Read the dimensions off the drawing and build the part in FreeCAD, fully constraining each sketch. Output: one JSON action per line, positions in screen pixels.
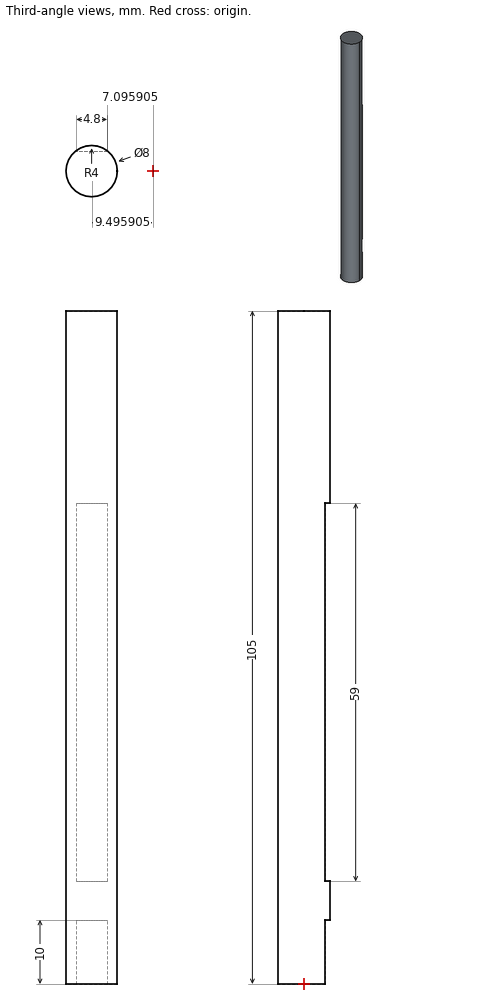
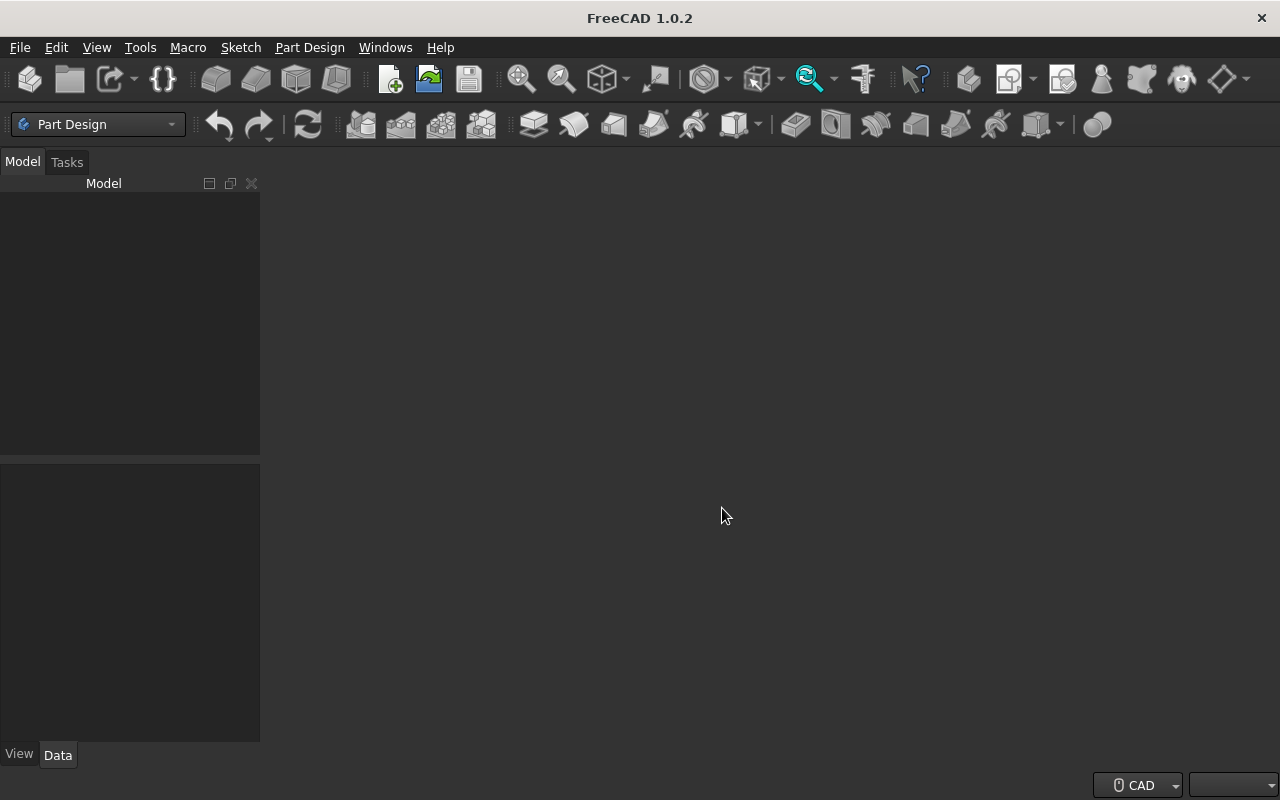
{"action": "left_click", "coordinate": [390, 80]}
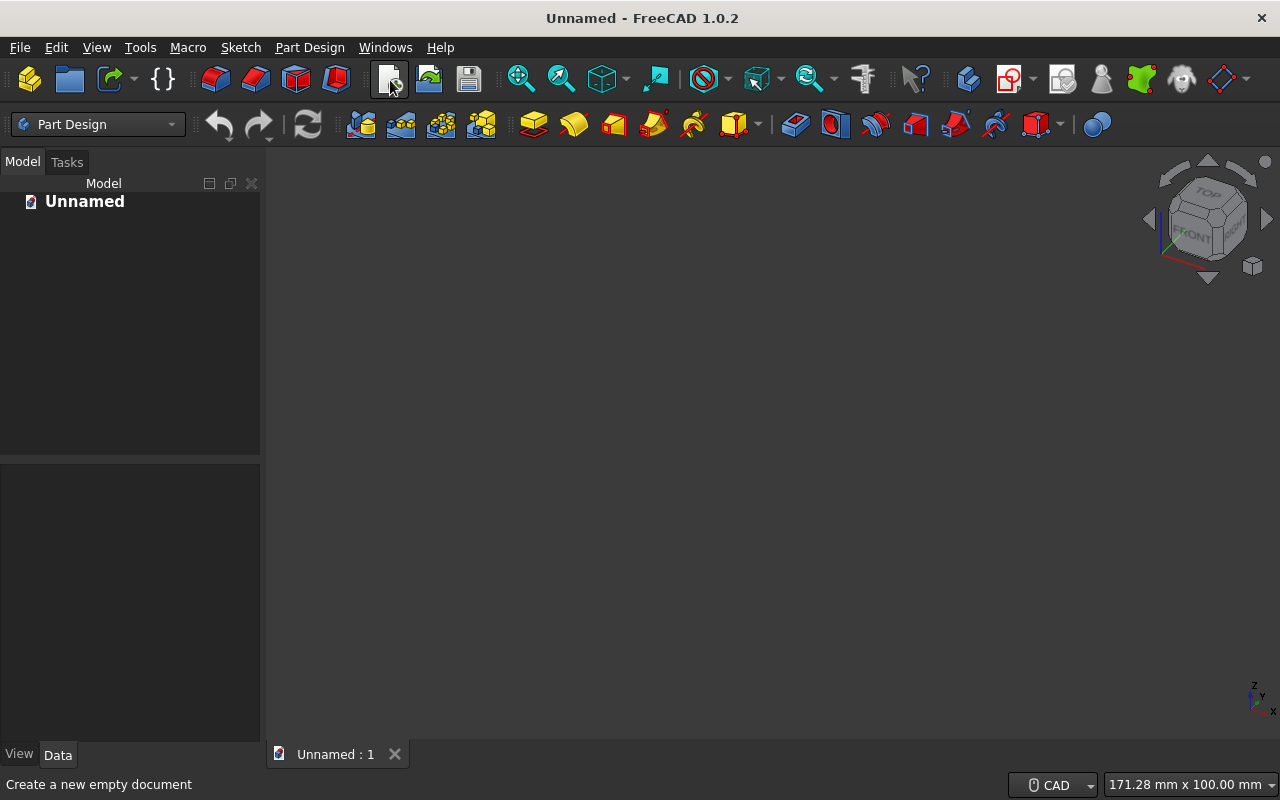
{"action": "left_click", "coordinate": [1010, 80]}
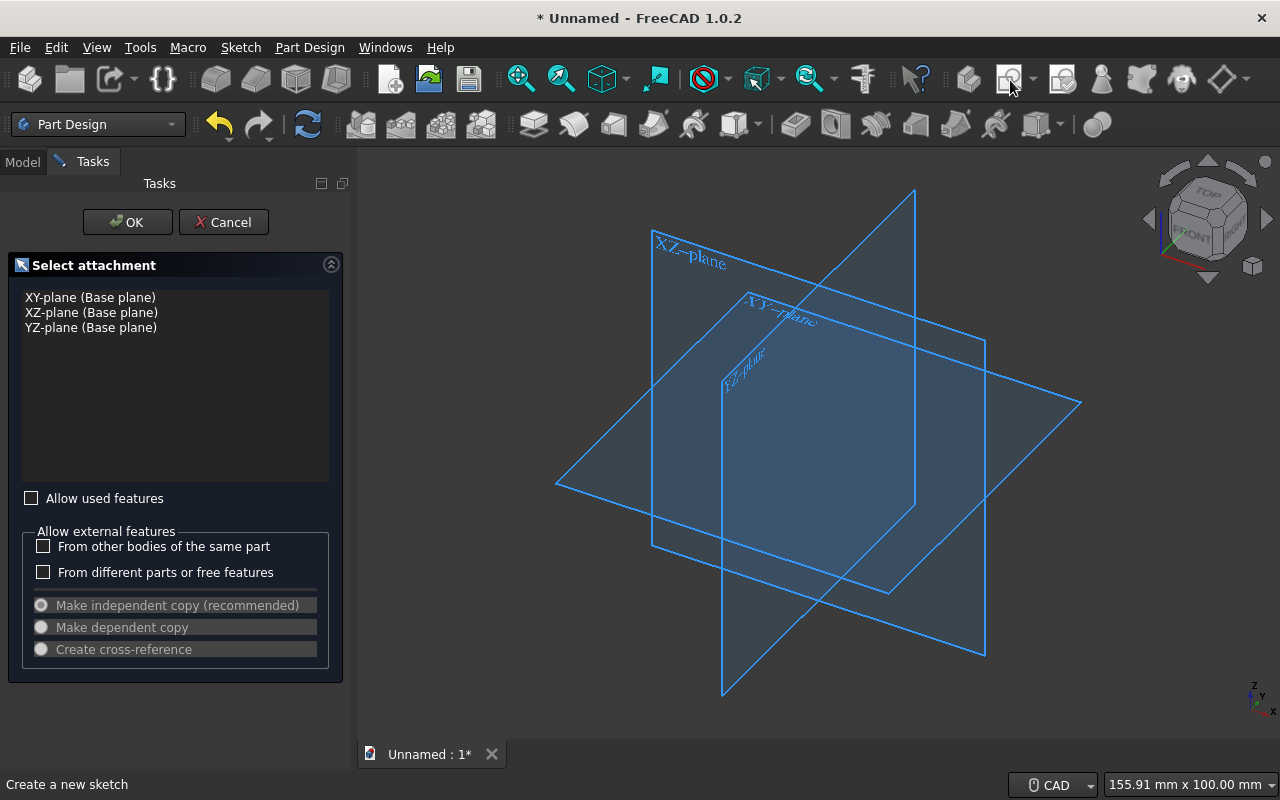
{"action": "left_click", "coordinate": [82, 298]}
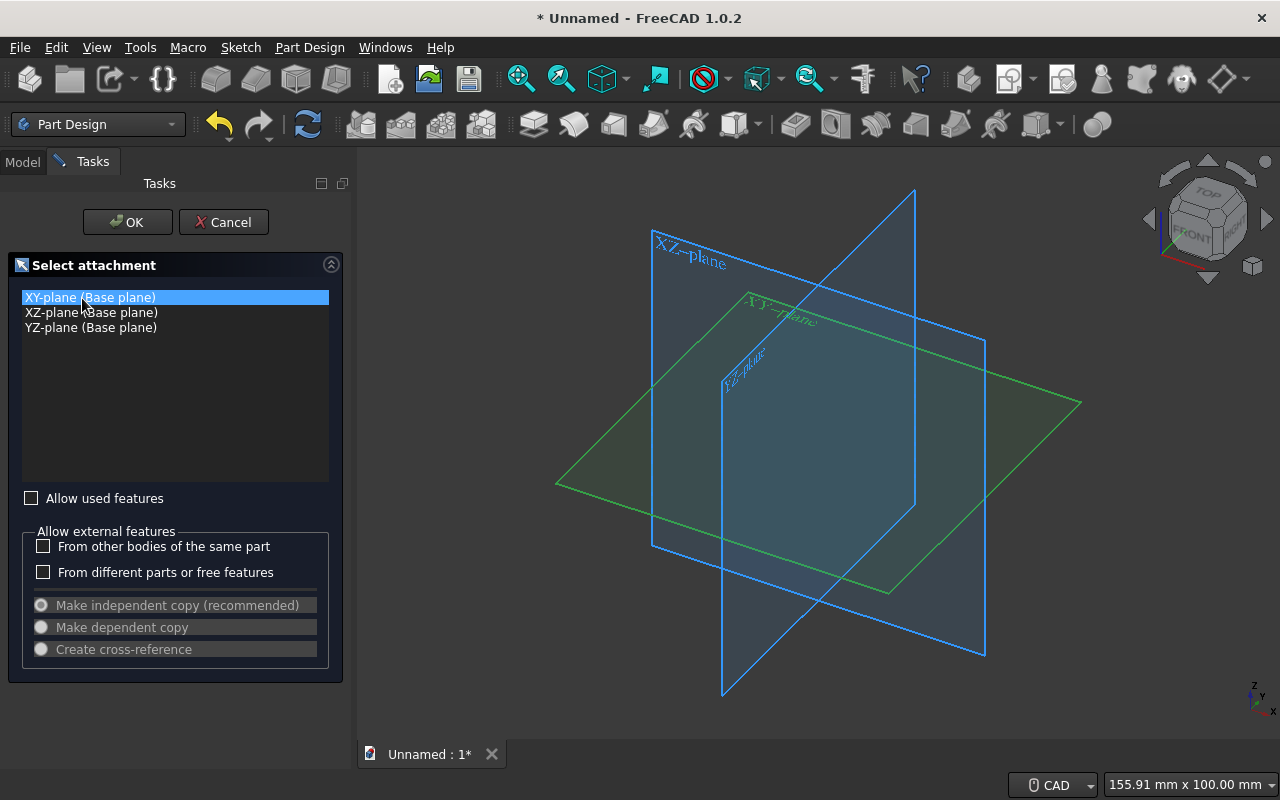
{"action": "left_click", "coordinate": [128, 222]}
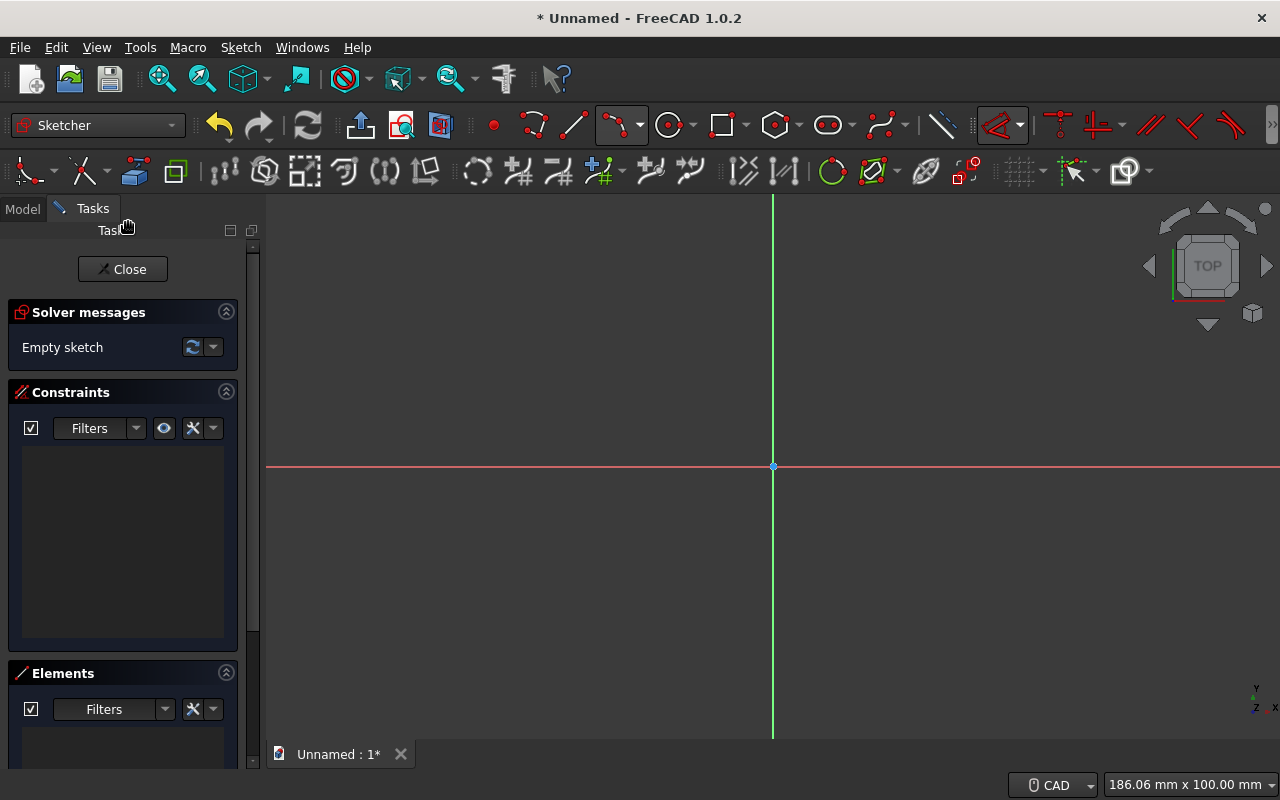
{"action": "scroll", "coordinate": [741, 466], "scroll_direction": "up", "scroll_amount": 10}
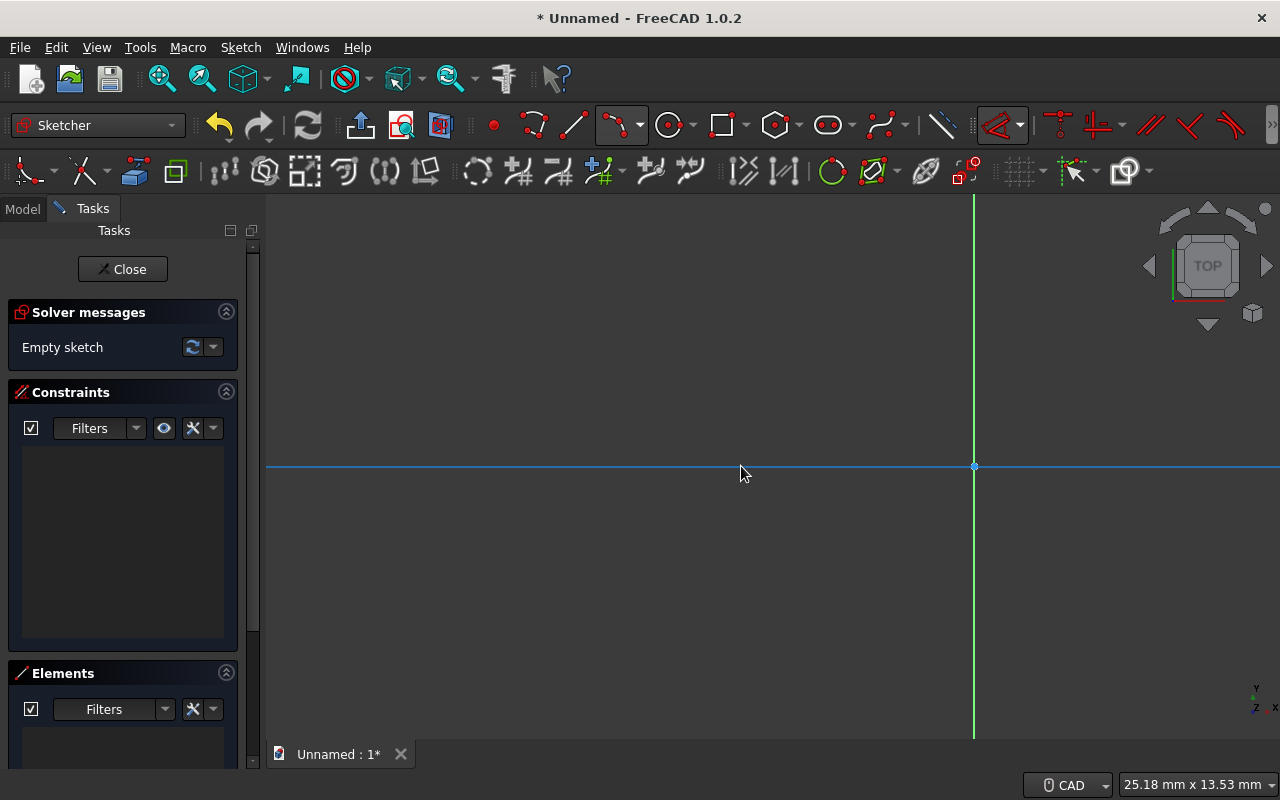
{"action": "key", "text": "g c"}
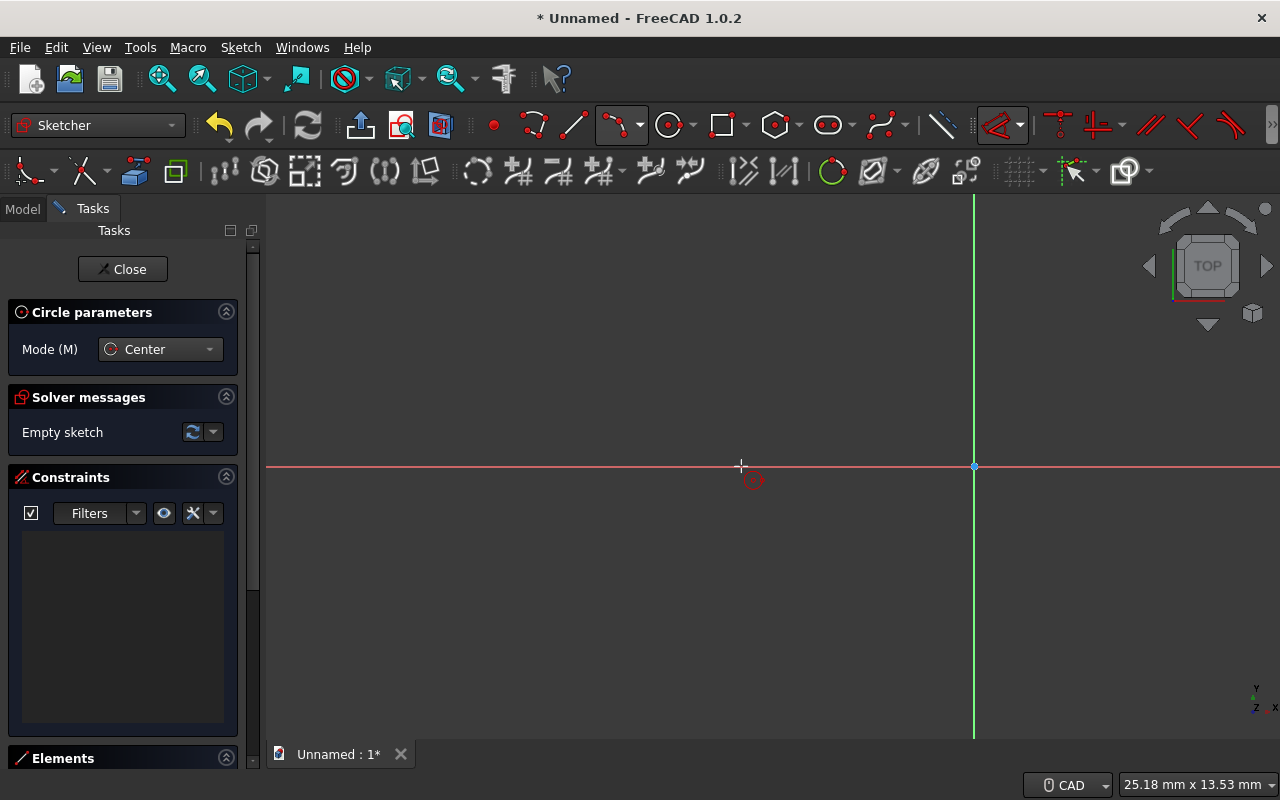
{"action": "left_click", "coordinate": [592, 466]}
{"action": "left_click", "coordinate": [706, 353]}
{"action": "key", "text": "Escape"}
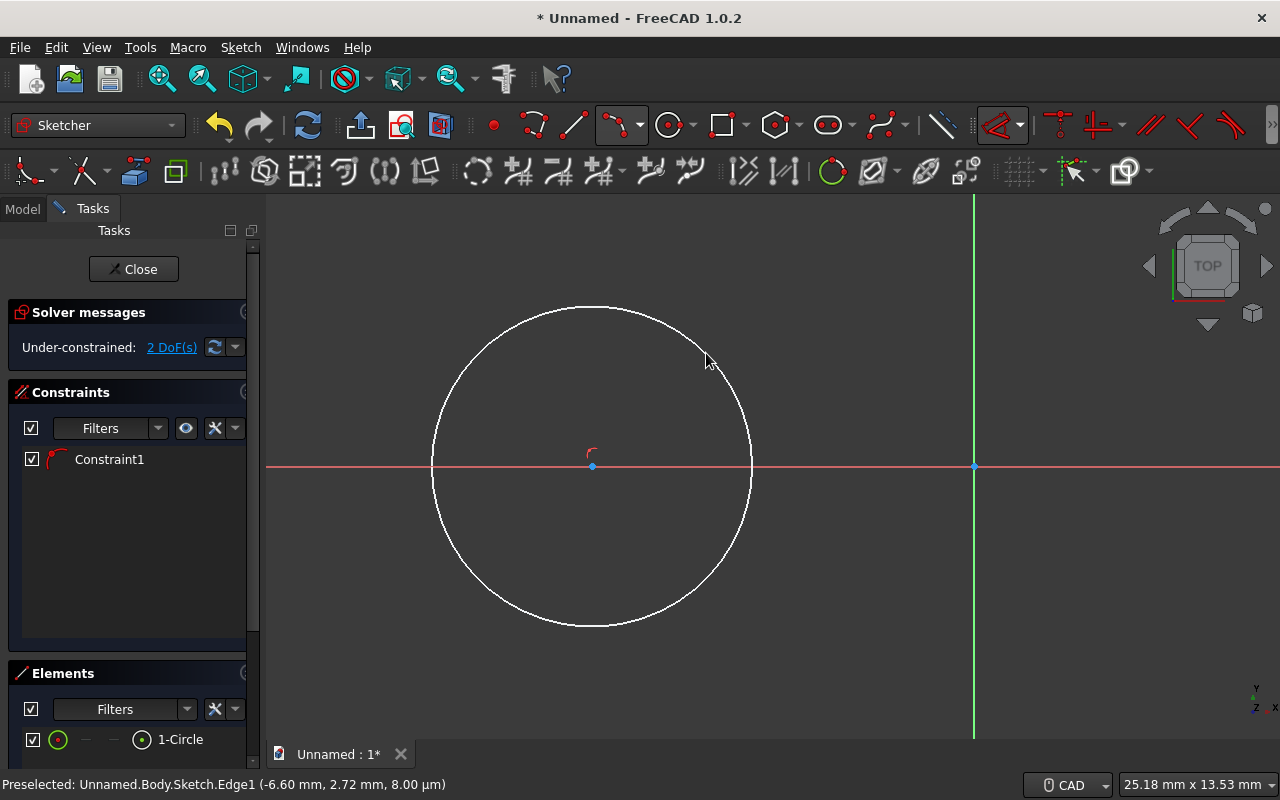
{"action": "left_click", "coordinate": [705, 353]}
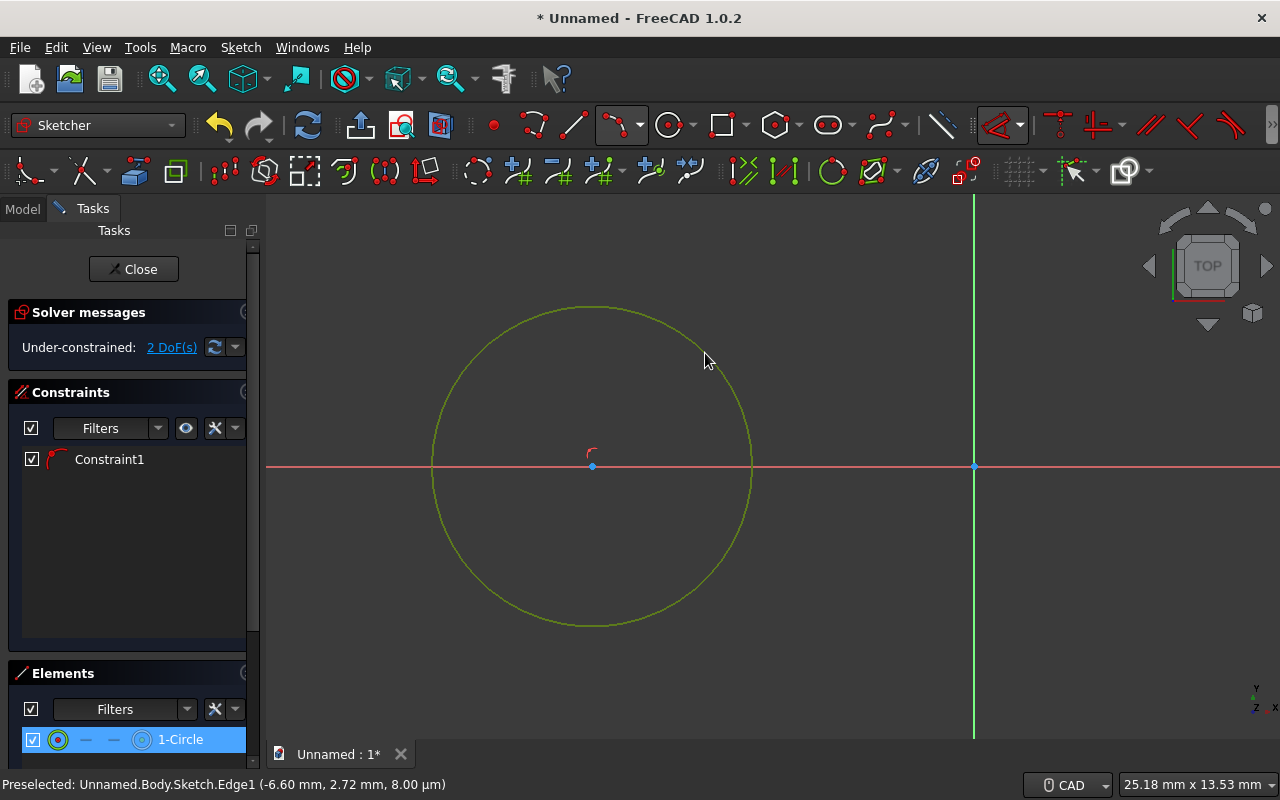
{"action": "key", "text": "k o"}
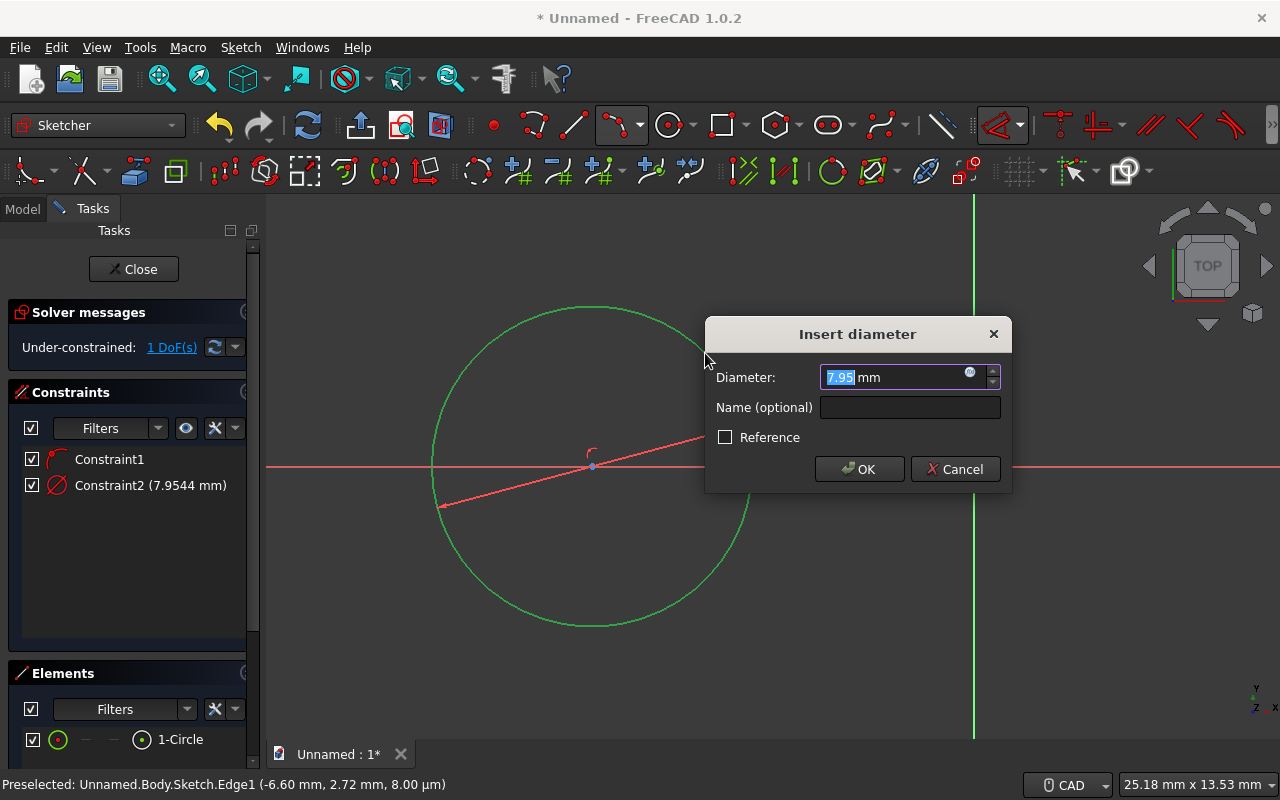
{"action": "type", "text": "8"}
{"action": "key", "text": "Return"}